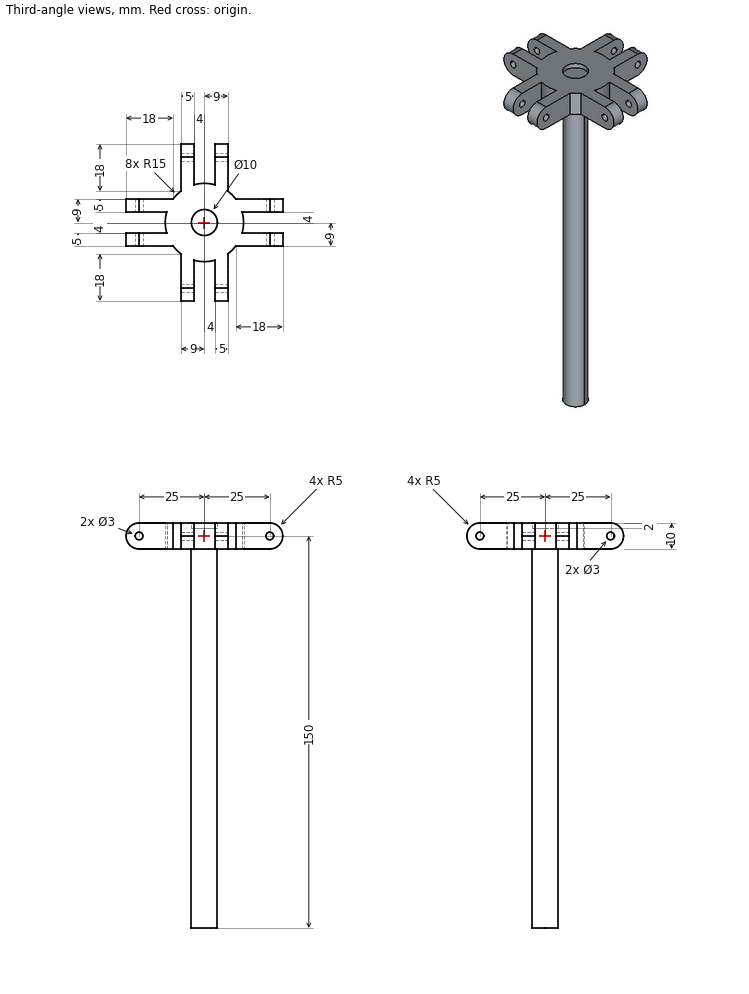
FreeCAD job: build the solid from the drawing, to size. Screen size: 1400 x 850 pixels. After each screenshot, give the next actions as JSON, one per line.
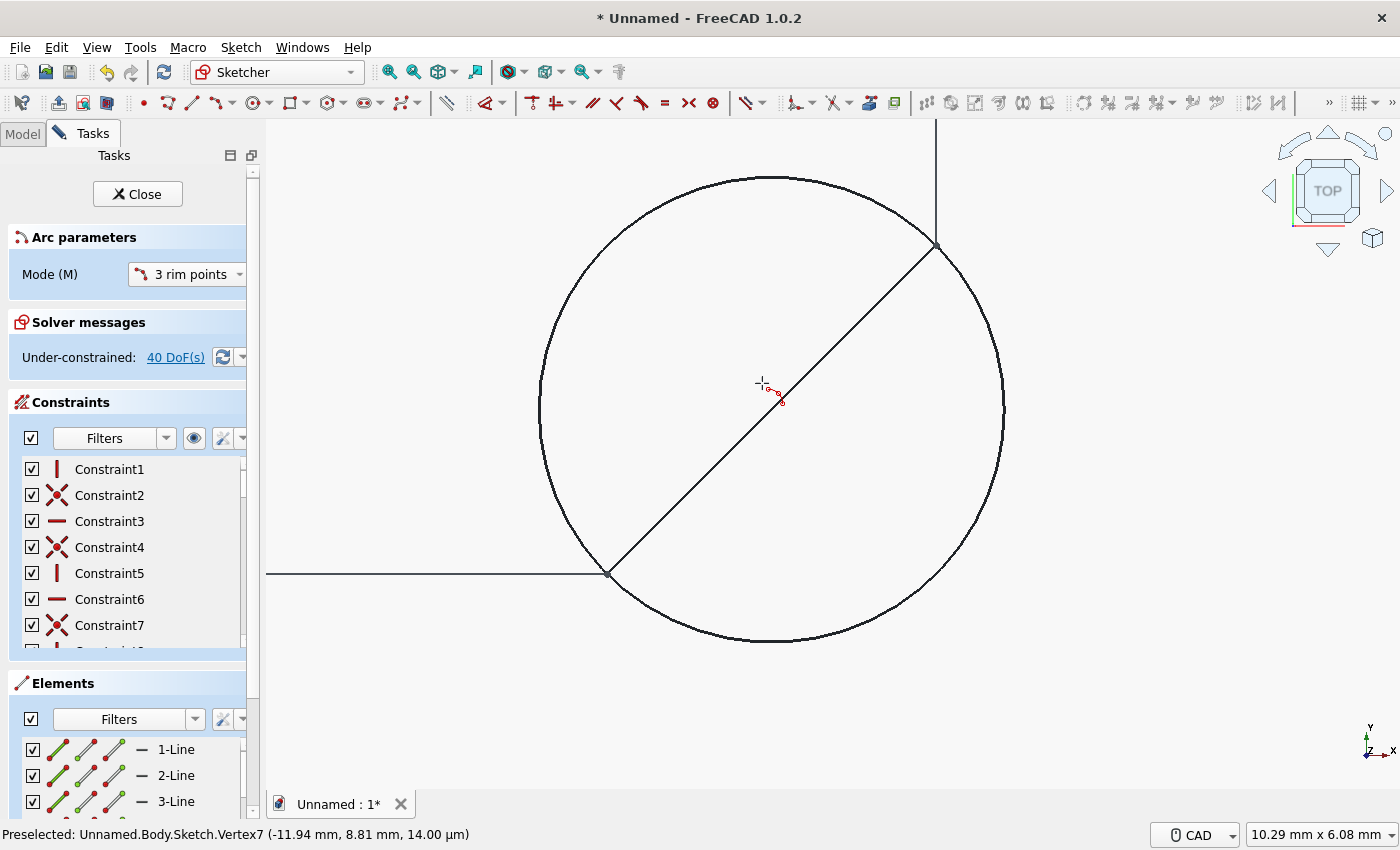
{"action": "left_click", "coordinate": [754, 376]}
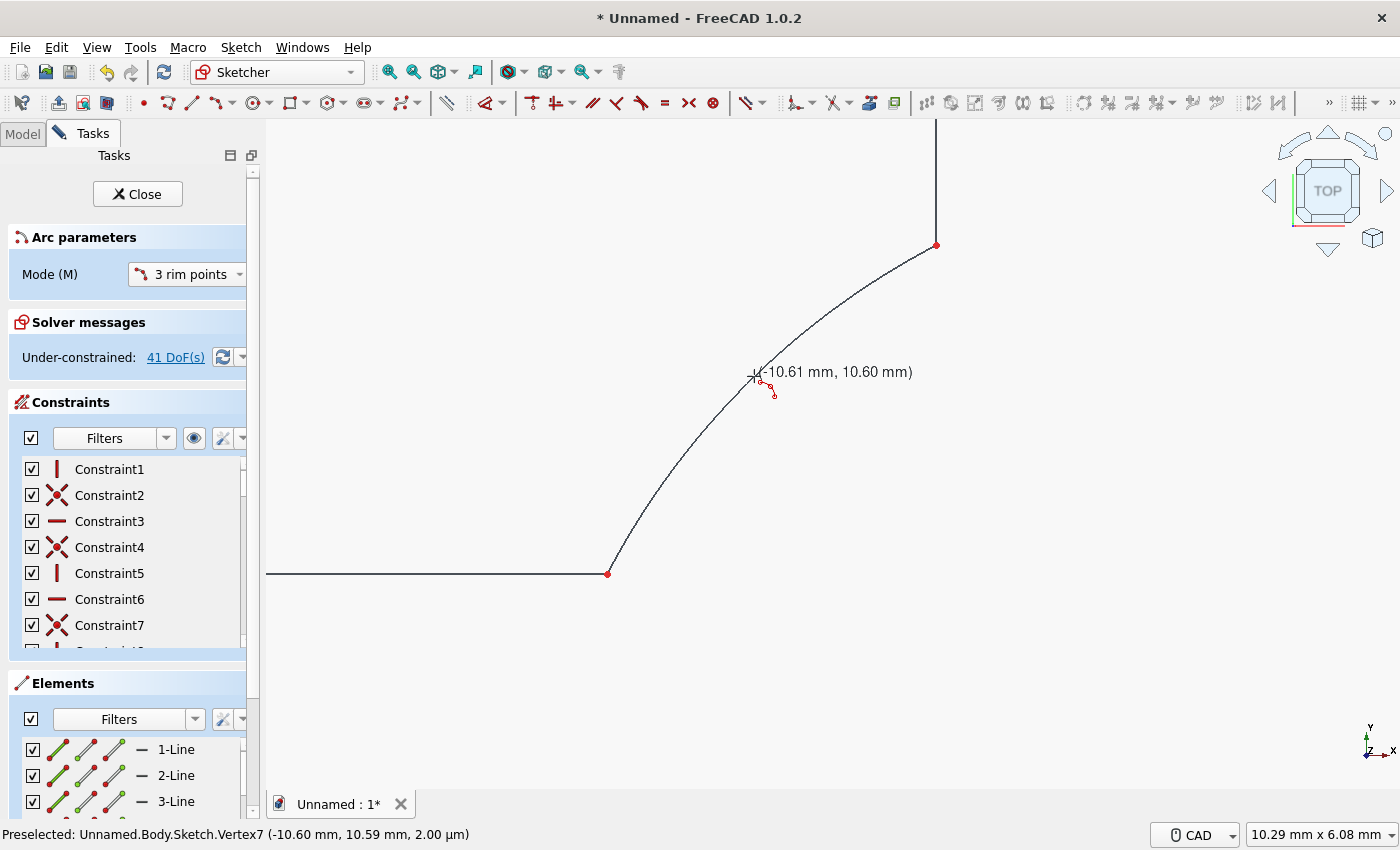
{"action": "scroll", "coordinate": [690, 383], "scroll_direction": "down", "scroll_amount": 14}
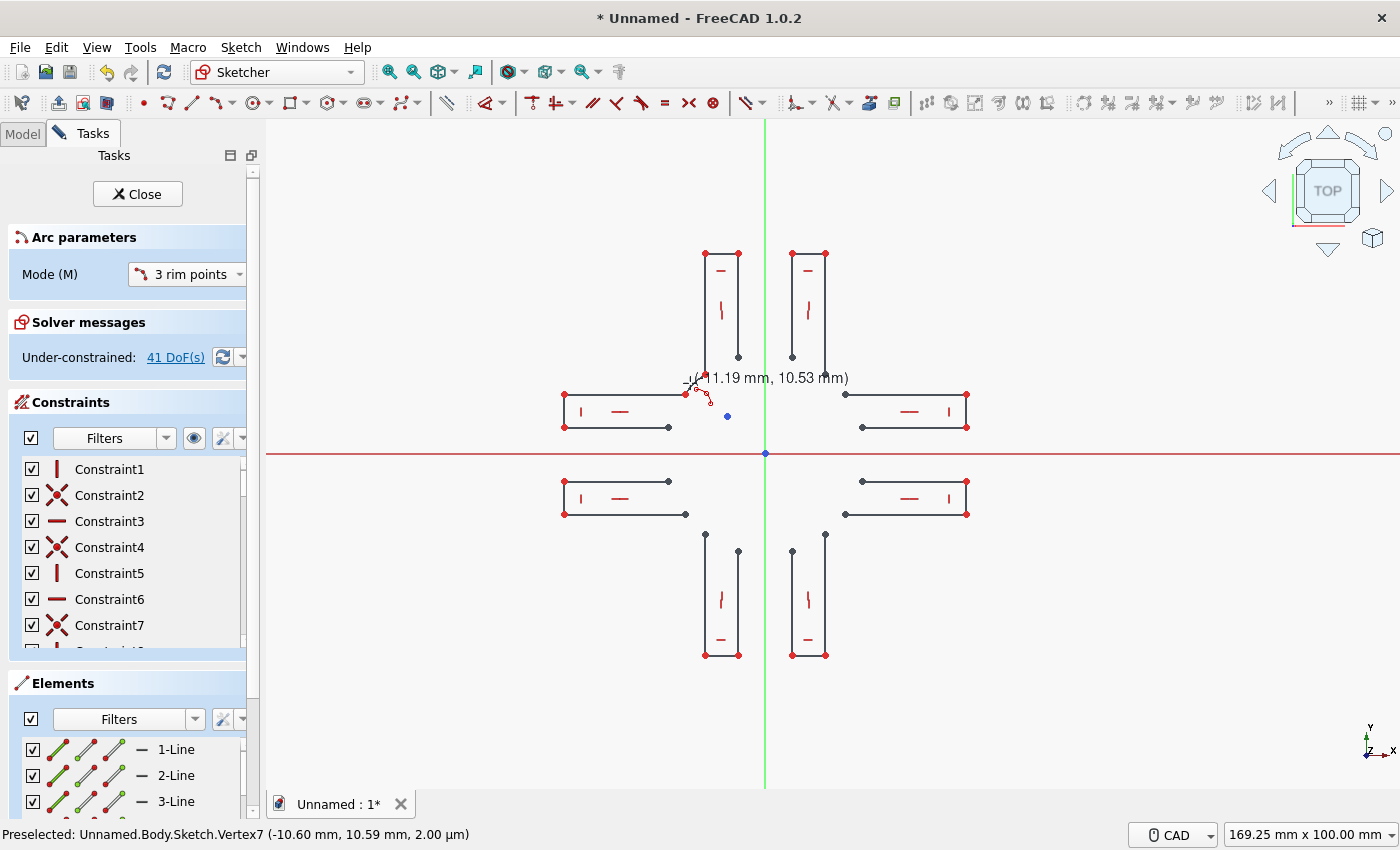
{"action": "left_click", "coordinate": [668, 428]}
{"action": "left_click", "coordinate": [668, 482]}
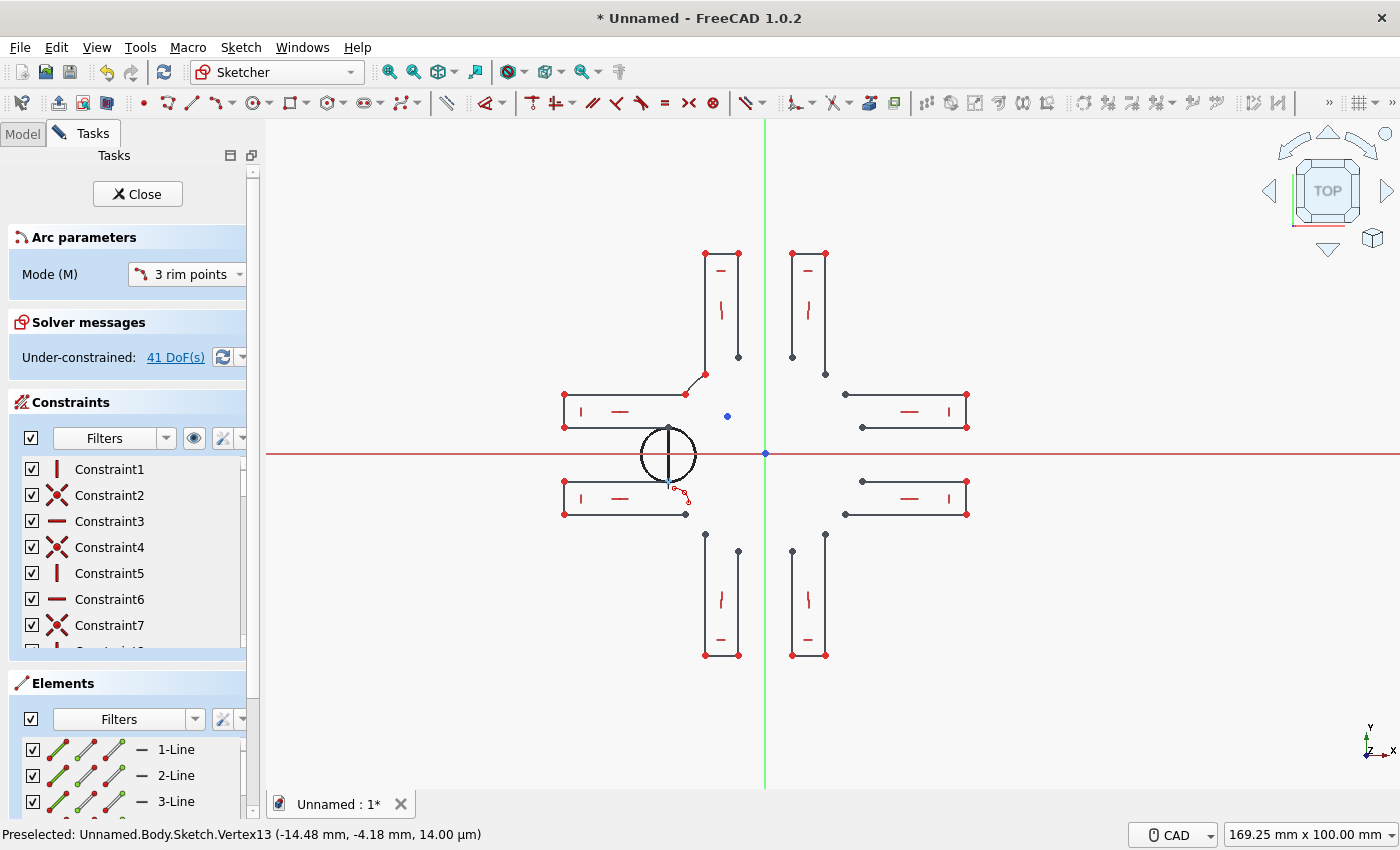
{"action": "scroll", "coordinate": [665, 459], "scroll_direction": "up", "scroll_amount": 8}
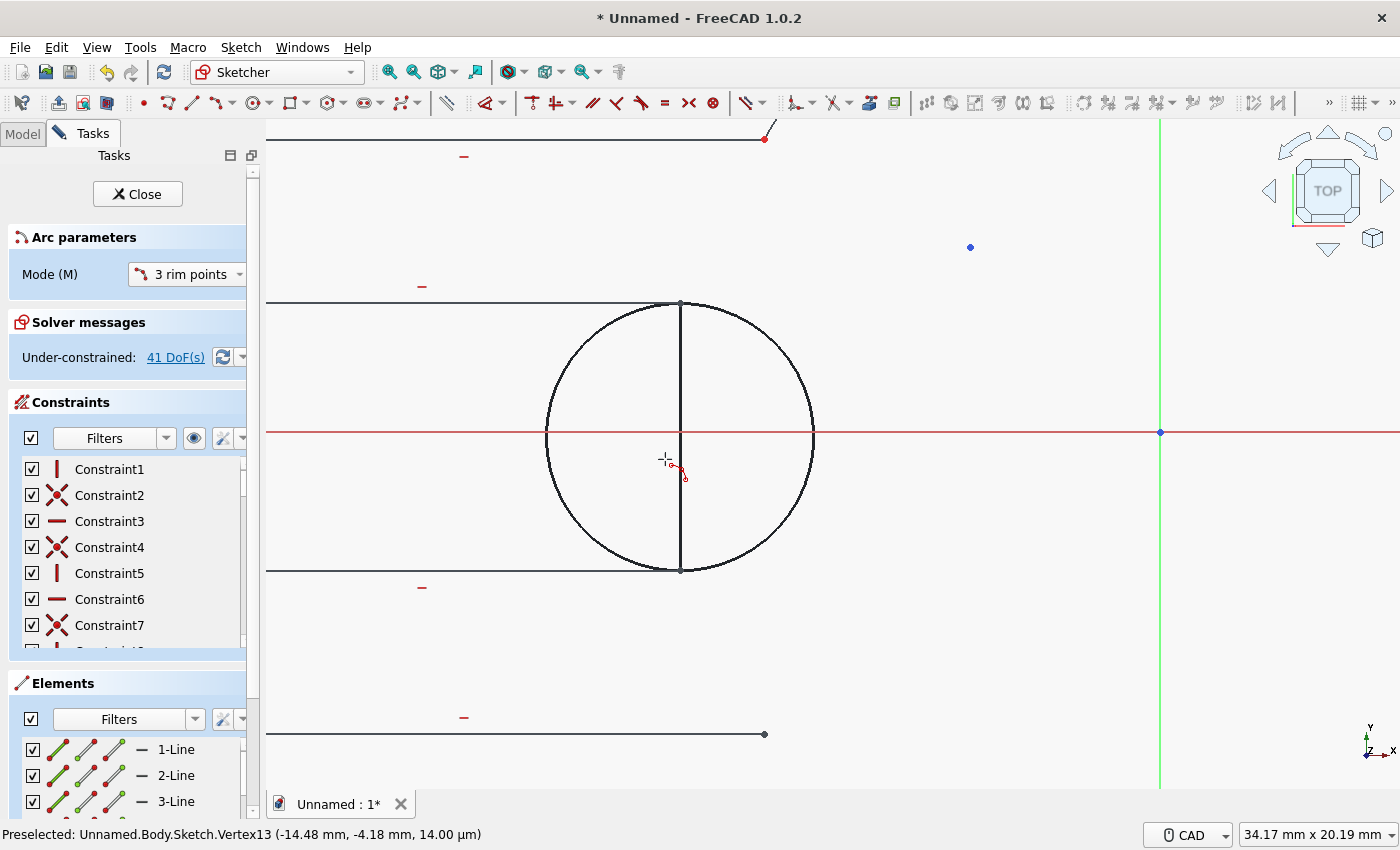
{"action": "left_click", "coordinate": [663, 459]}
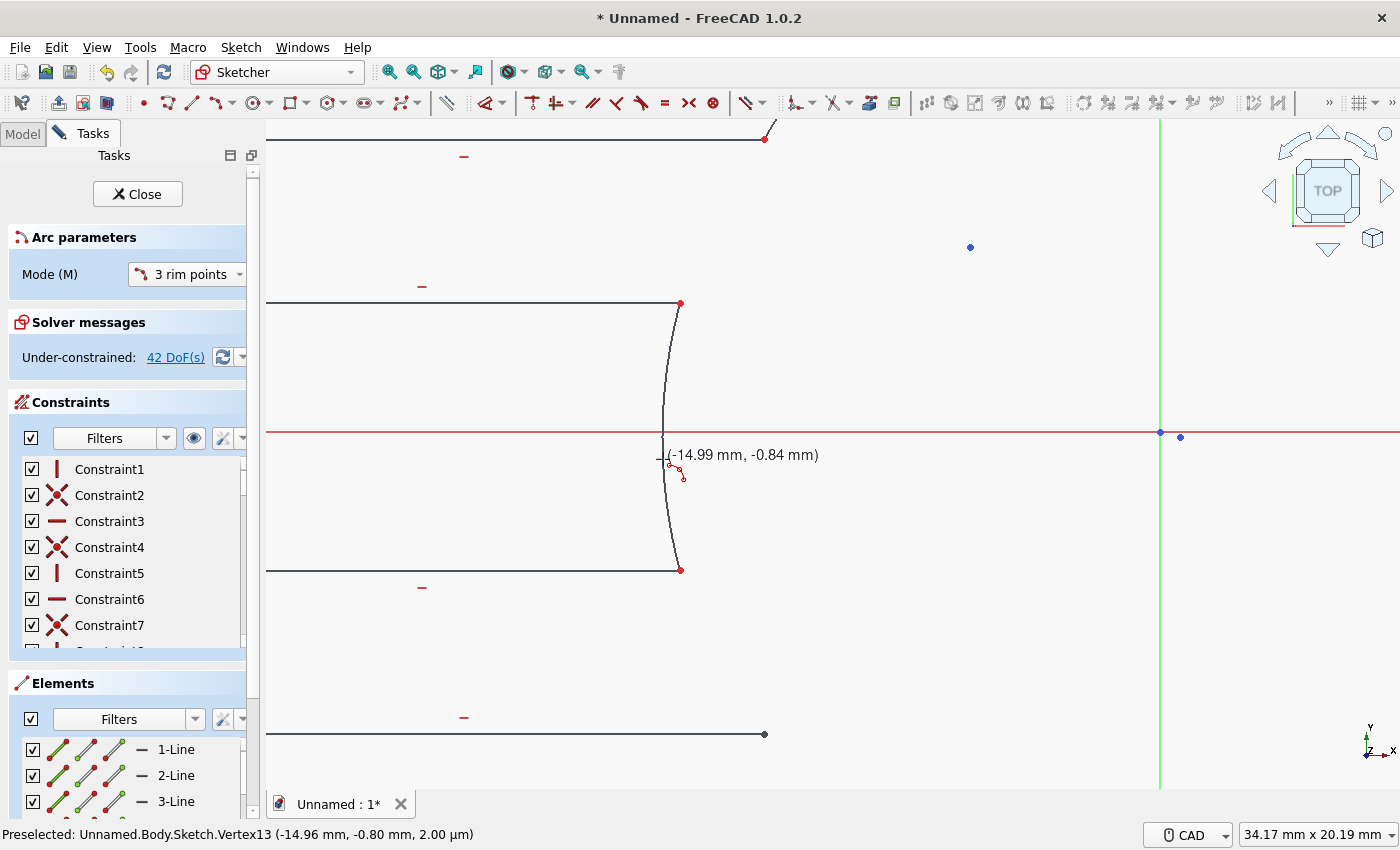
{"action": "scroll", "coordinate": [664, 460], "scroll_direction": "down", "scroll_amount": 8}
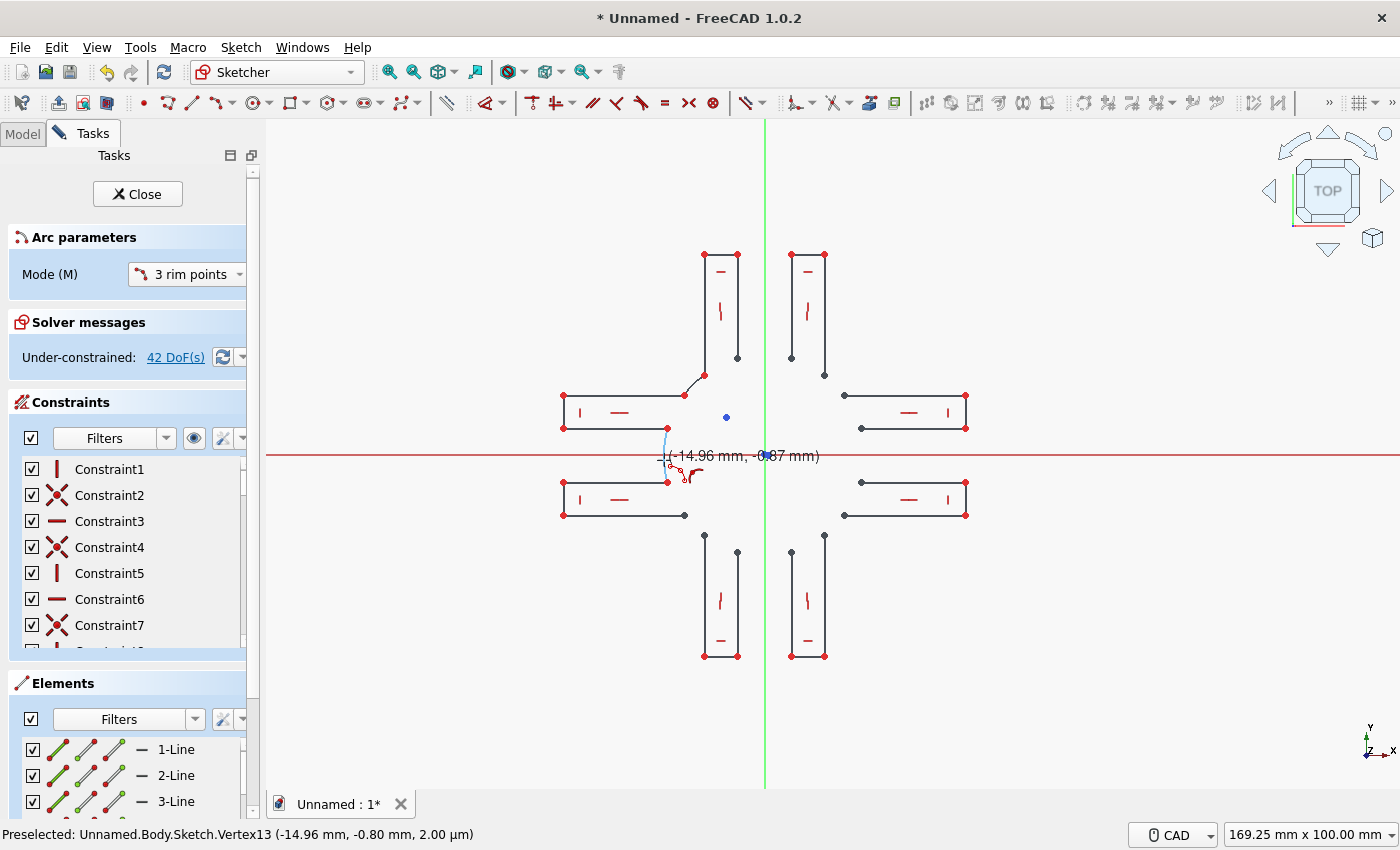
{"action": "left_click", "coordinate": [685, 516]}
{"action": "left_click", "coordinate": [705, 536]}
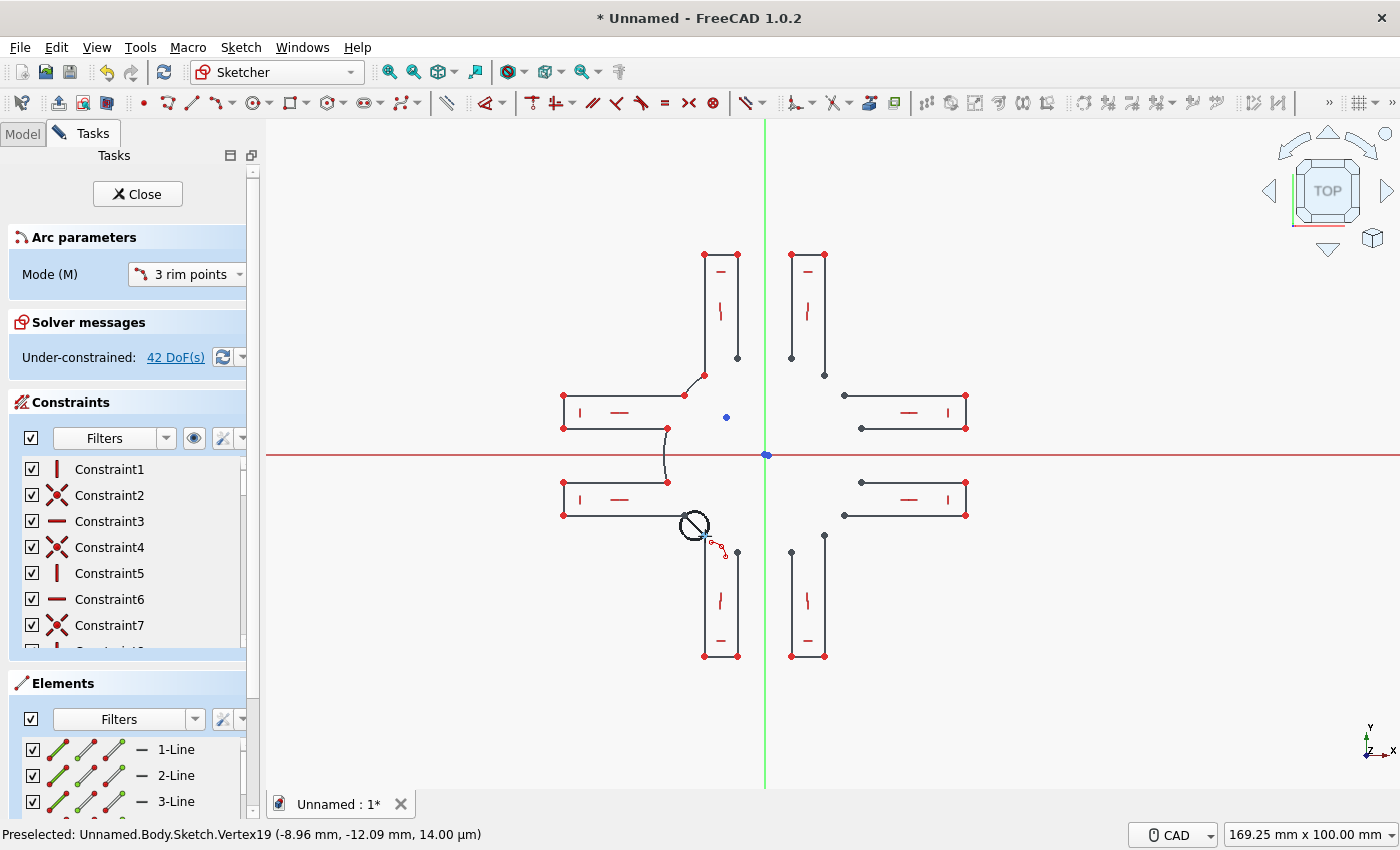
{"action": "scroll", "coordinate": [693, 526], "scroll_direction": "up", "scroll_amount": 14}